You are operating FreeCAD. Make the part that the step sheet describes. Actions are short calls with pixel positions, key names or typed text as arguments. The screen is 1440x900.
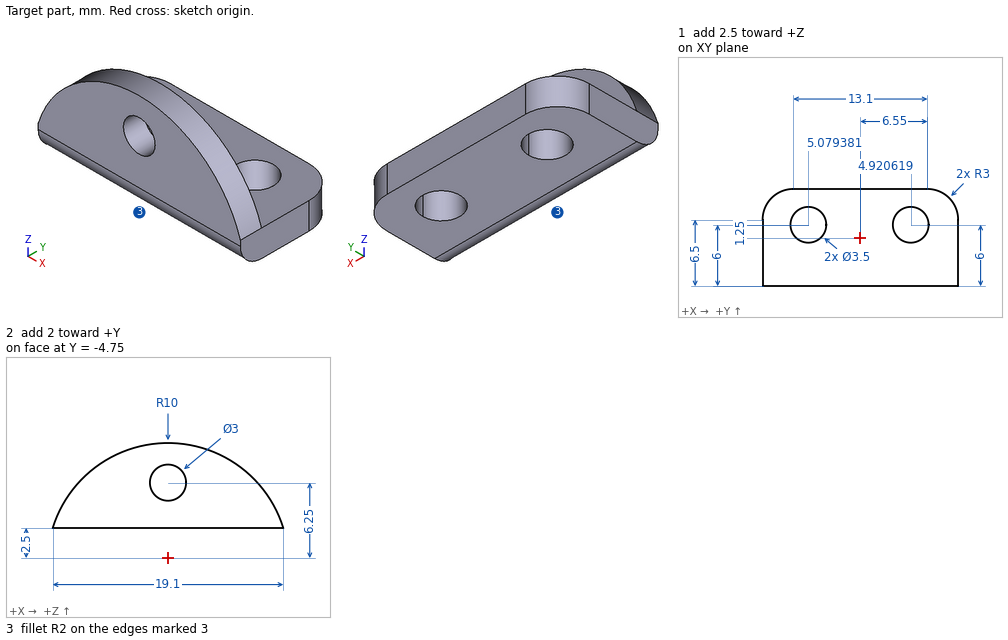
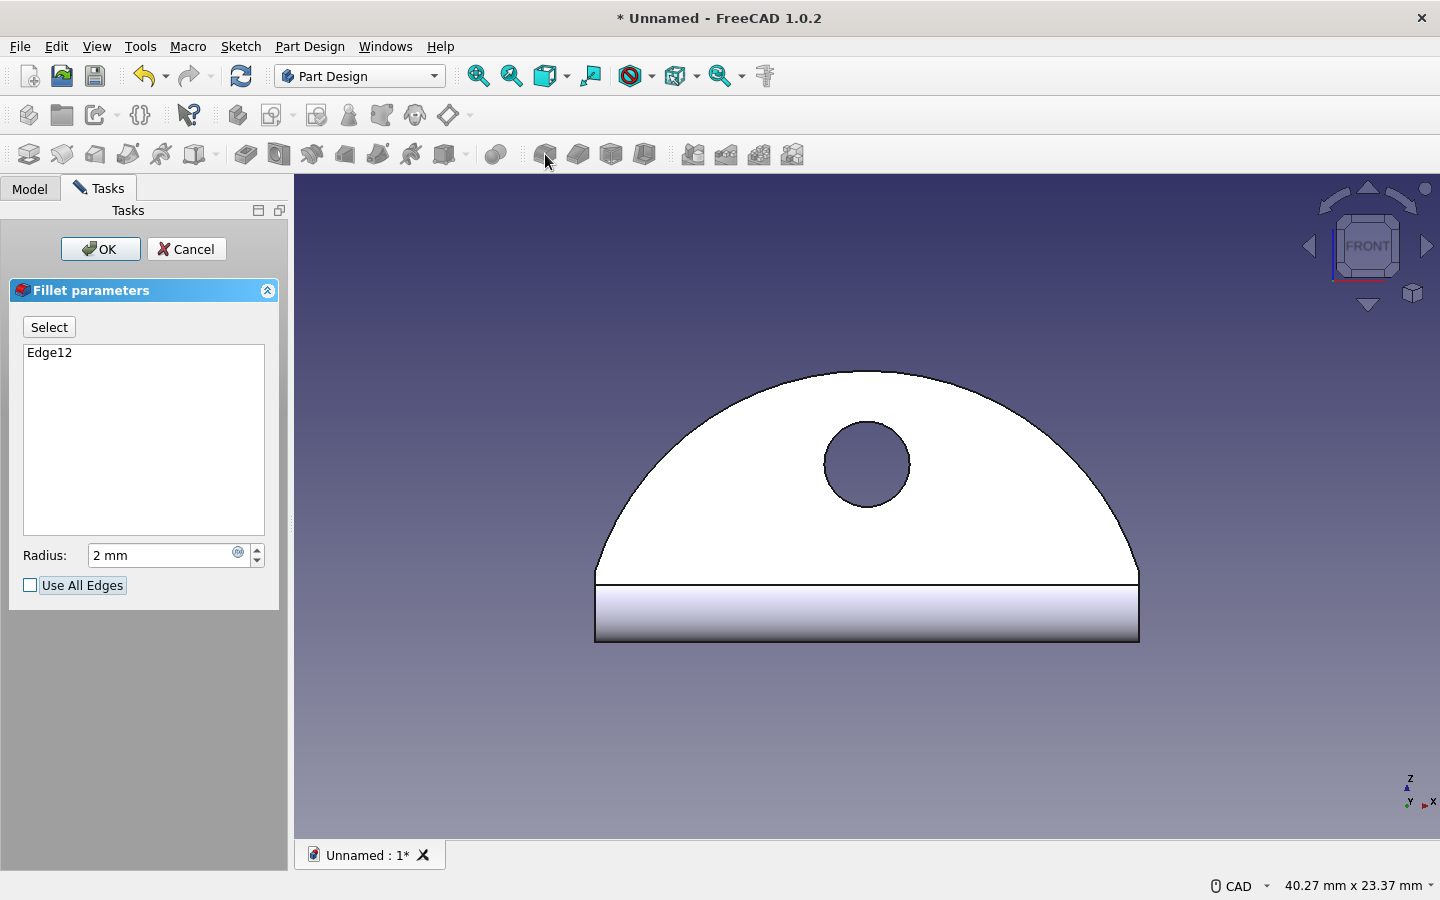
click(101, 249)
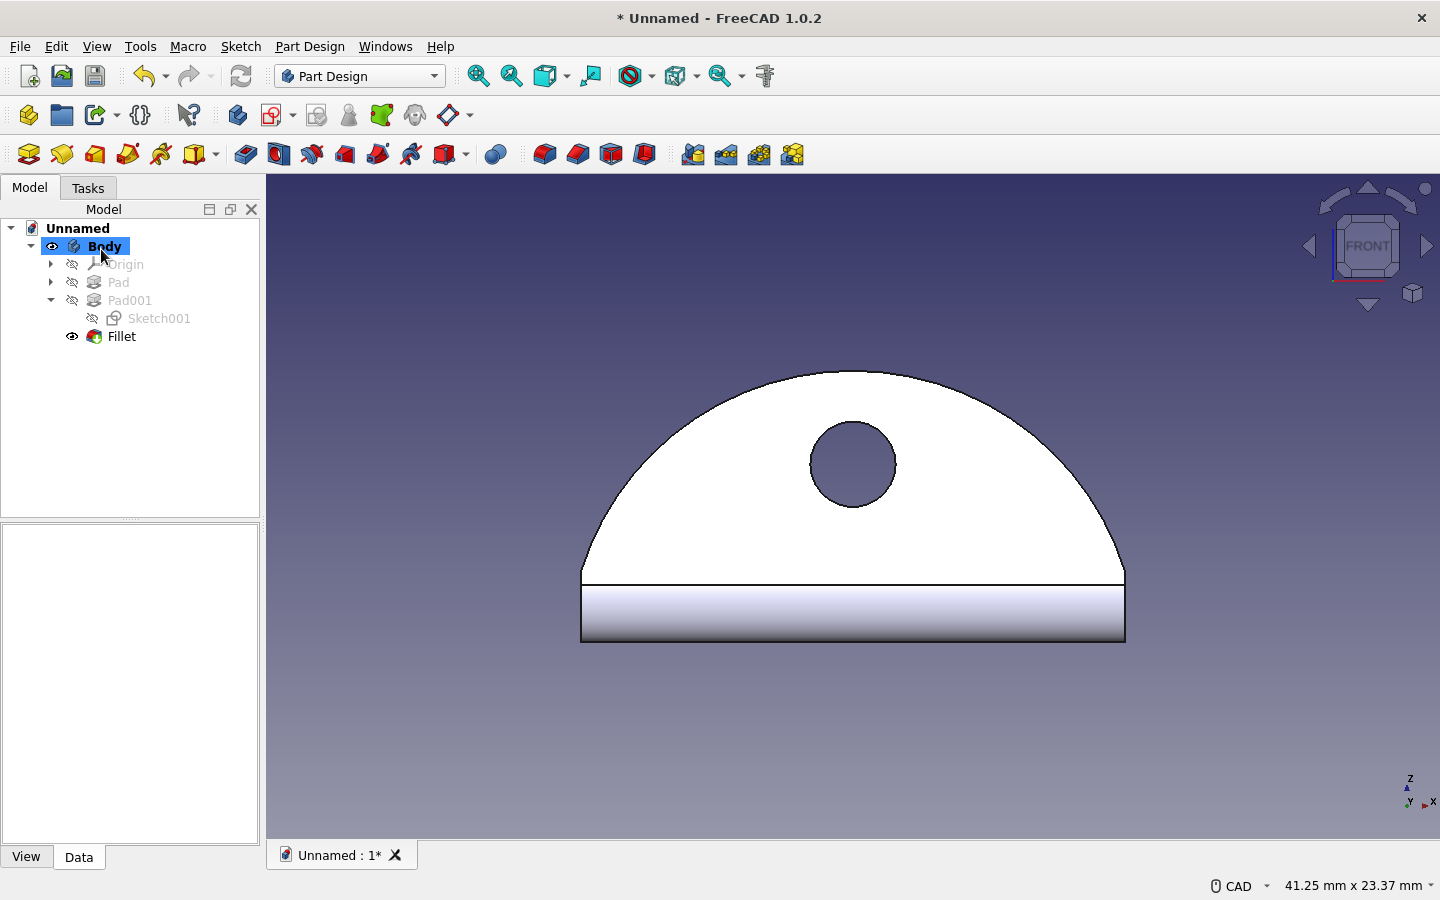
key(0)